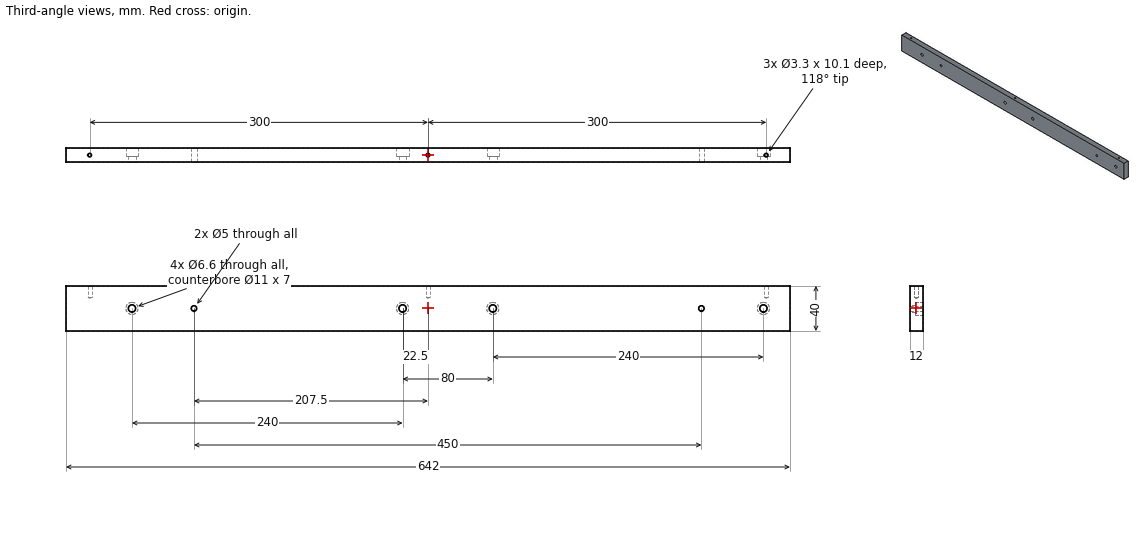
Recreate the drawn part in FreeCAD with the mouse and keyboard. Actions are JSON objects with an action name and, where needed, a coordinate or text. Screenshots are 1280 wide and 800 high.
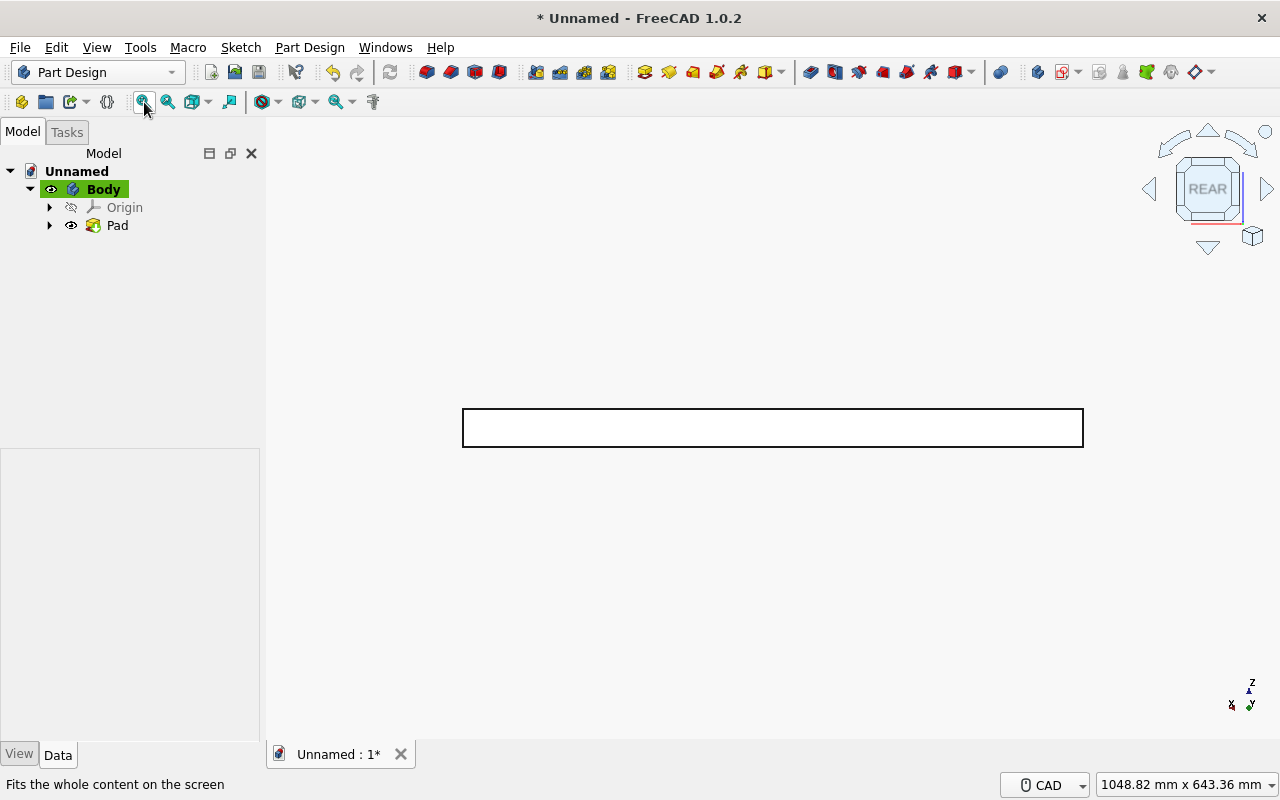
{"action": "left_click", "coordinate": [507, 427]}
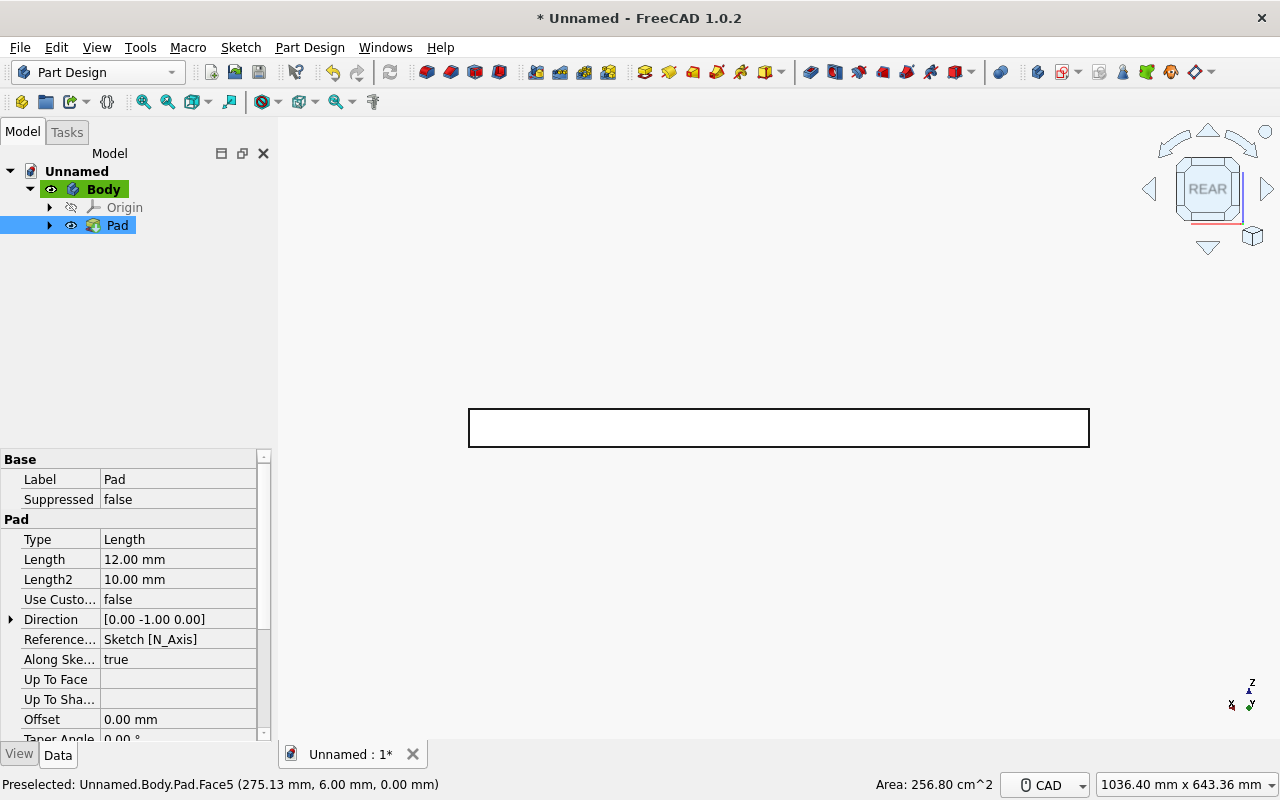
{"action": "left_click", "coordinate": [1062, 72]}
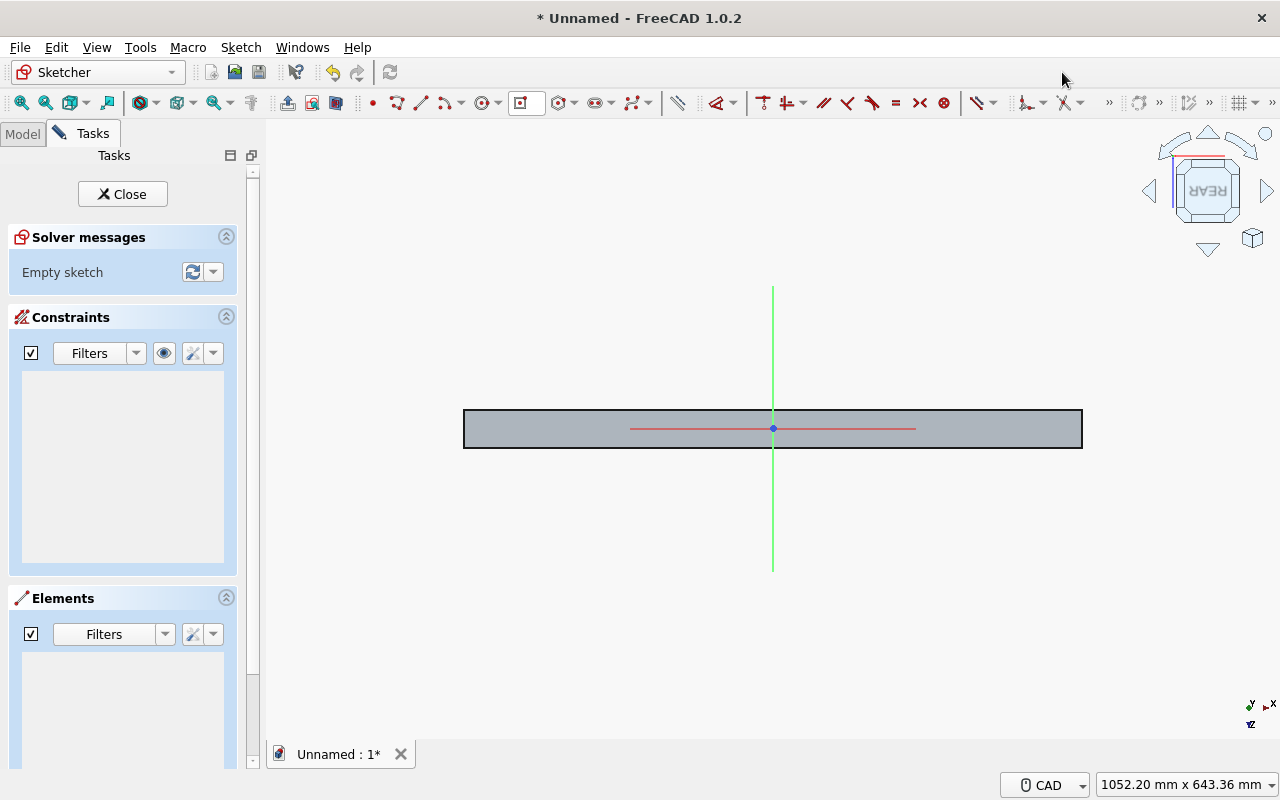
{"action": "left_click", "coordinate": [482, 104]}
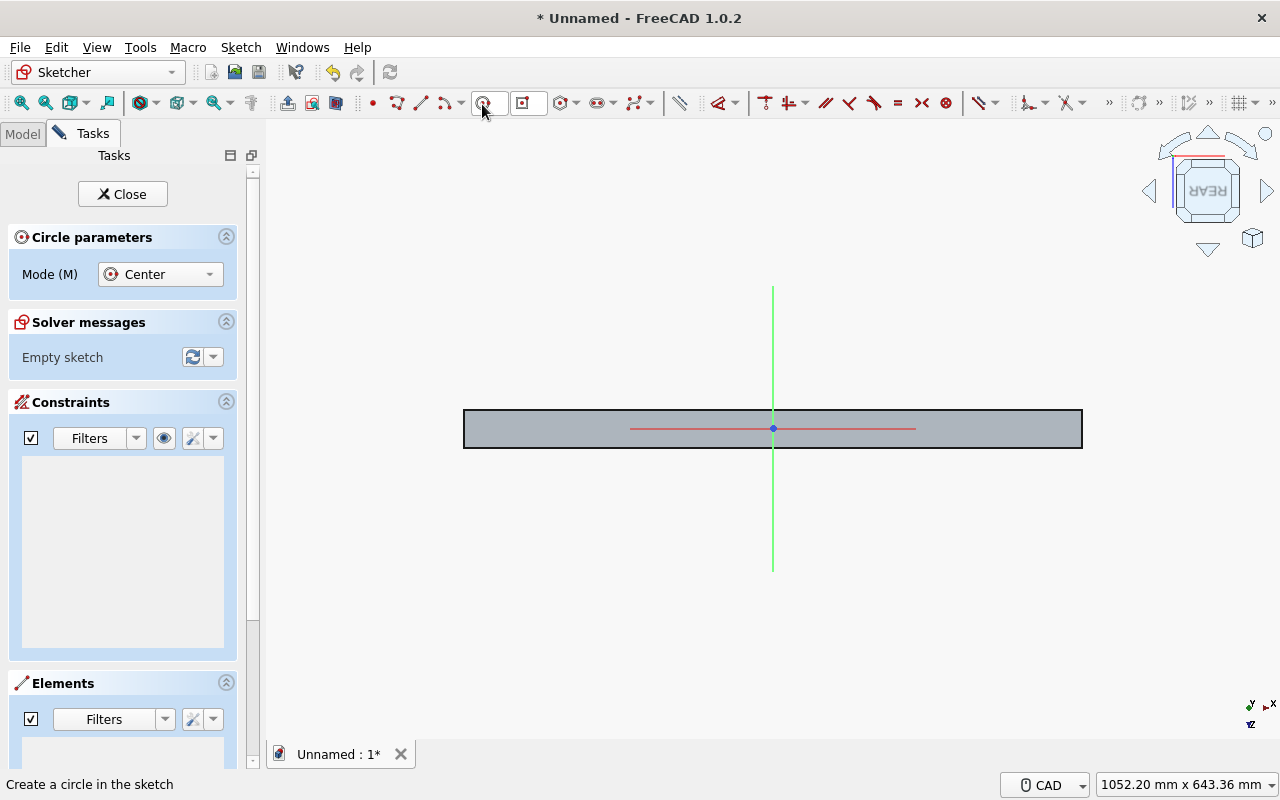
{"action": "scroll", "coordinate": [520, 429], "scroll_direction": "up", "scroll_amount": 10}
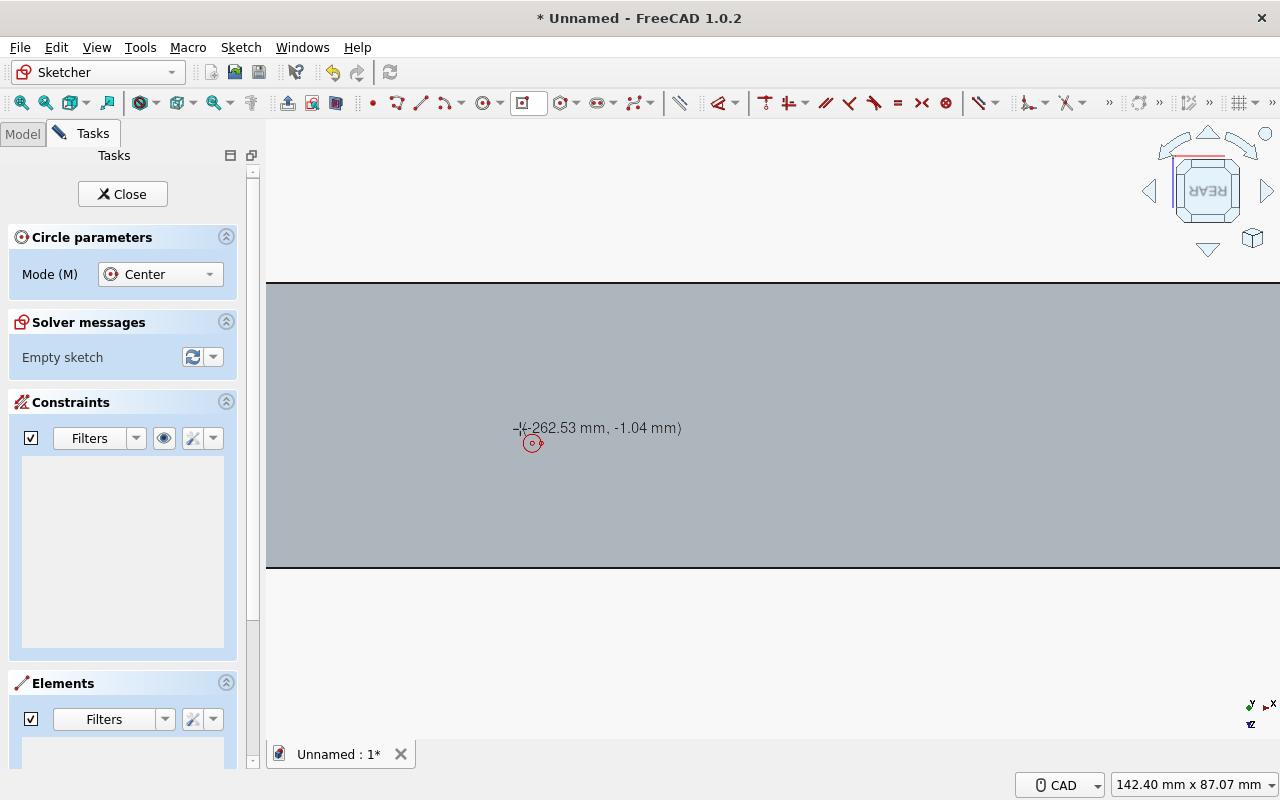
{"action": "scroll", "coordinate": [422, 430], "scroll_direction": "down", "scroll_amount": 10}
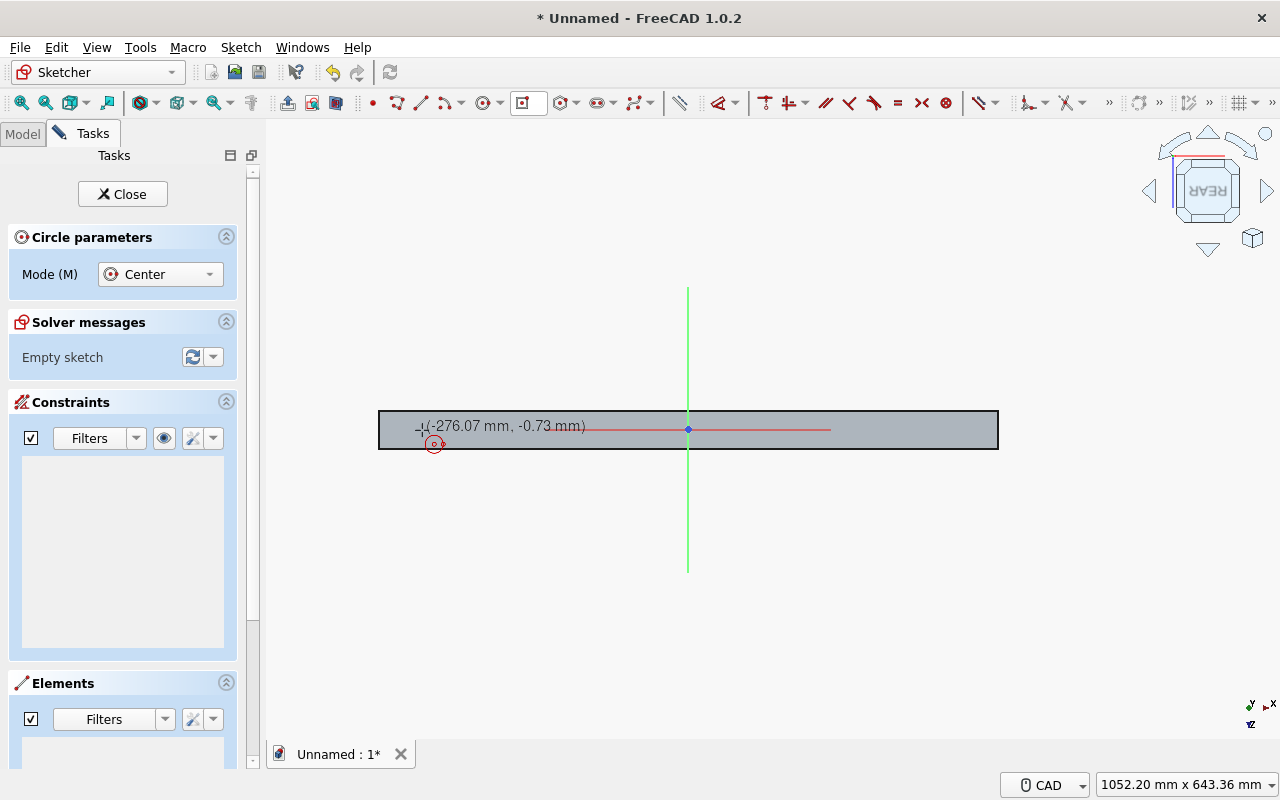
{"action": "left_click", "coordinate": [435, 430]}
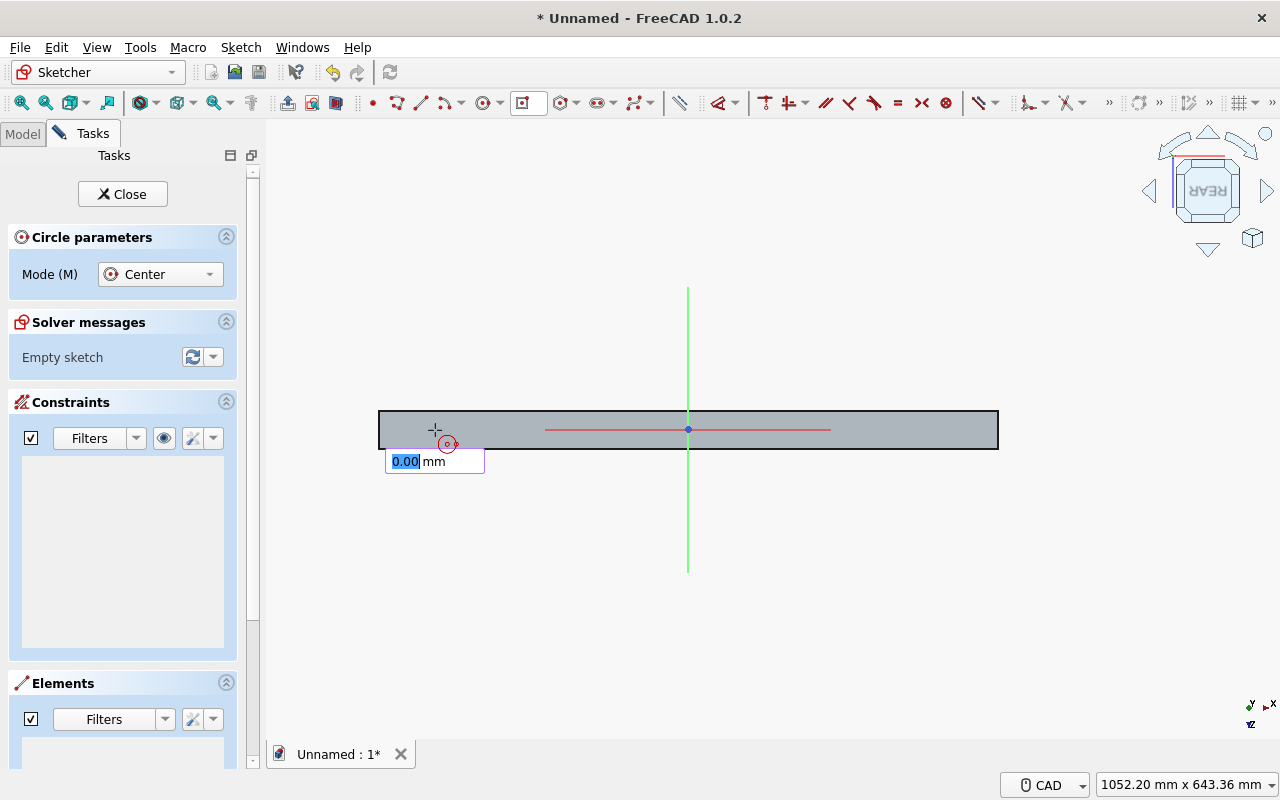
{"action": "scroll", "coordinate": [434, 433], "scroll_direction": "up", "scroll_amount": 9}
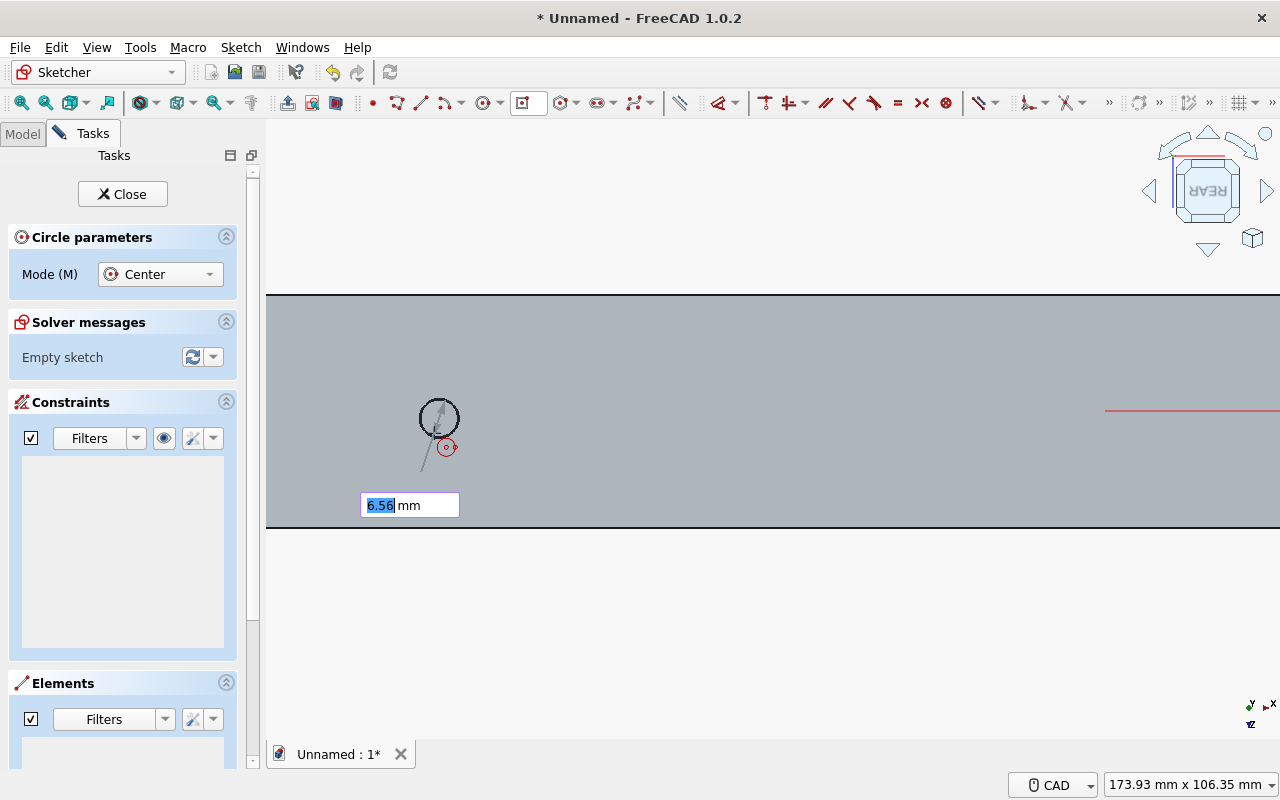
{"action": "left_click", "coordinate": [434, 430]}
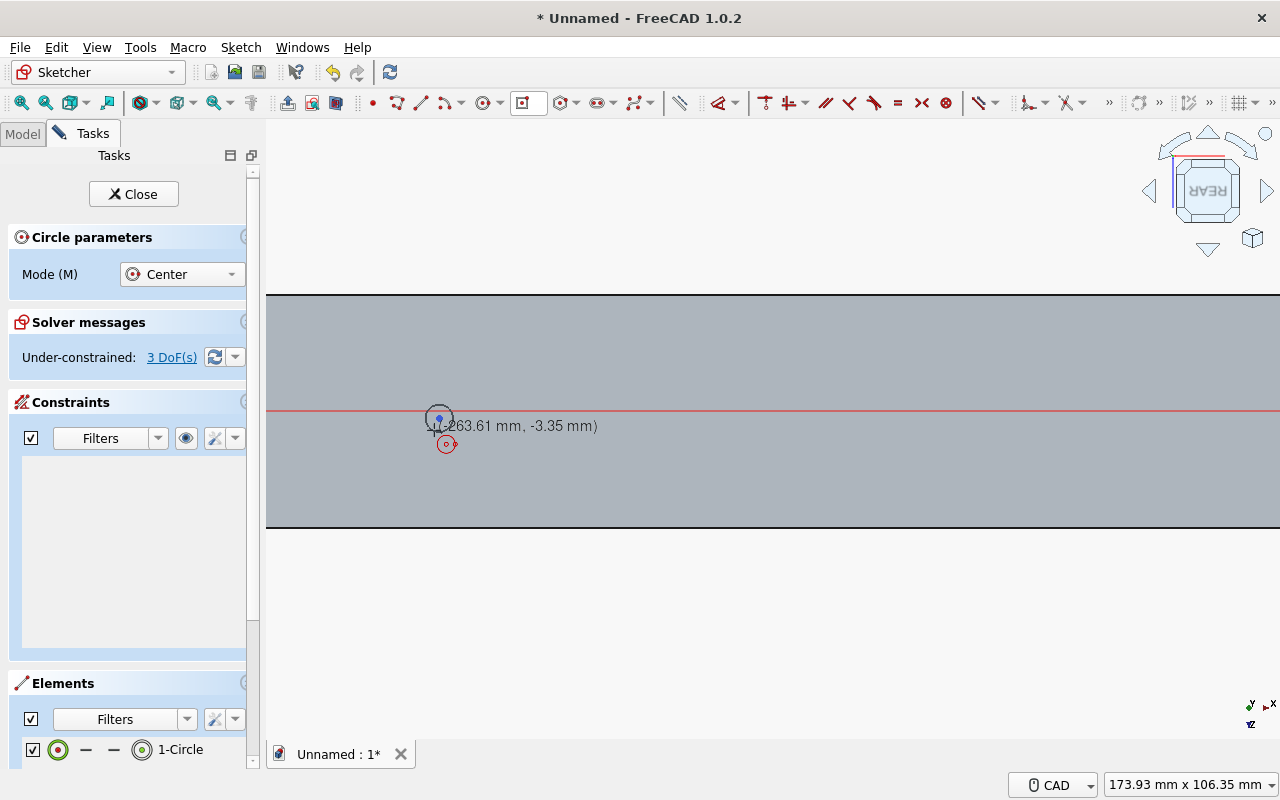
{"action": "scroll", "coordinate": [434, 432], "scroll_direction": "down", "scroll_amount": 9}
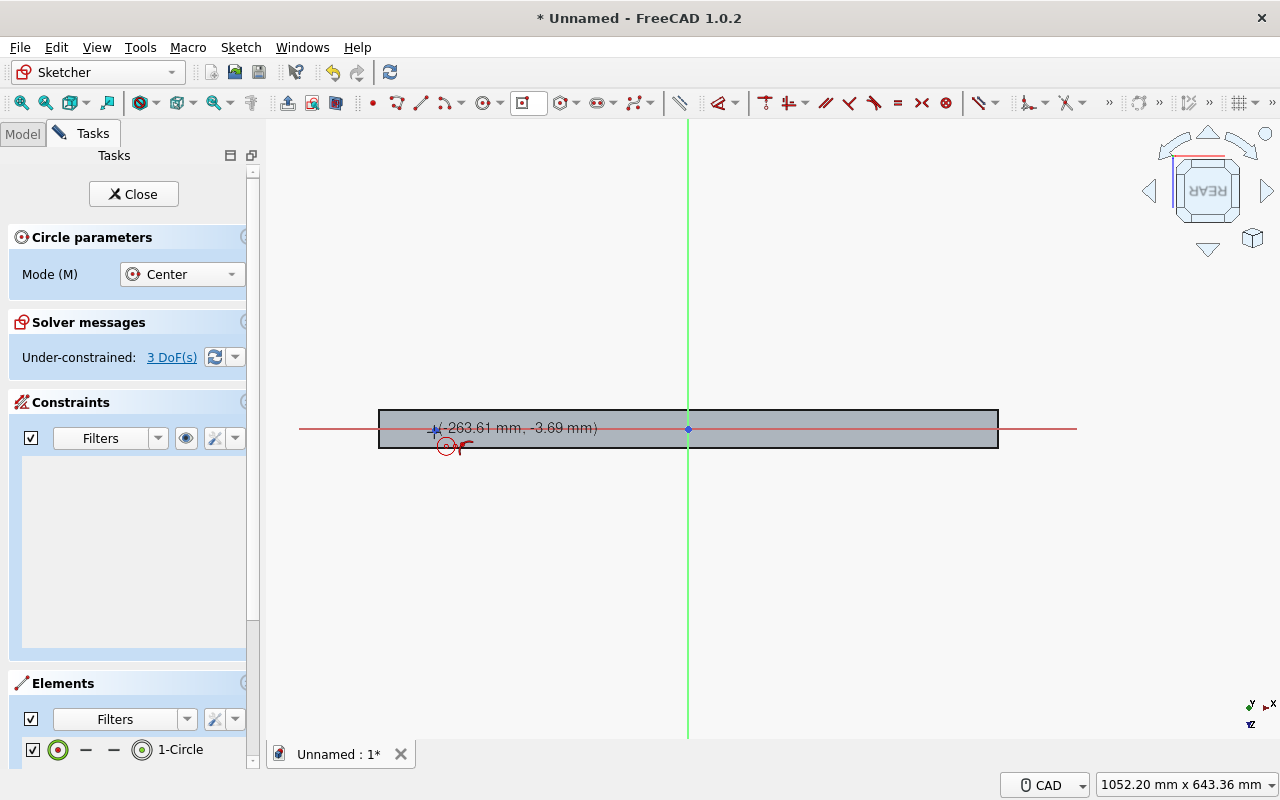
{"action": "scroll", "coordinate": [666, 429], "scroll_direction": "up", "scroll_amount": 10}